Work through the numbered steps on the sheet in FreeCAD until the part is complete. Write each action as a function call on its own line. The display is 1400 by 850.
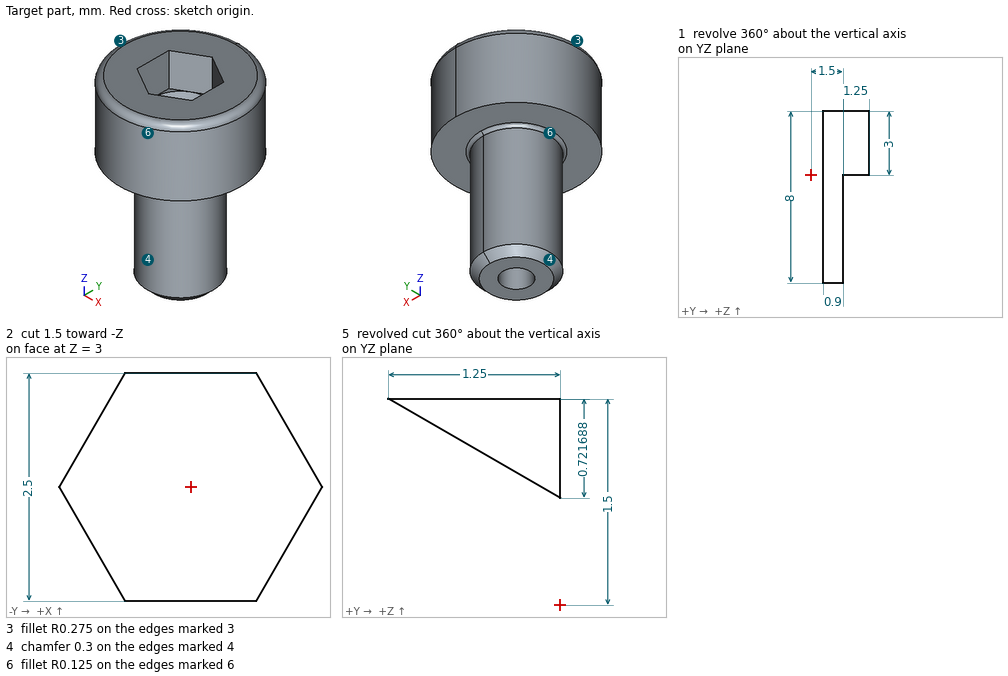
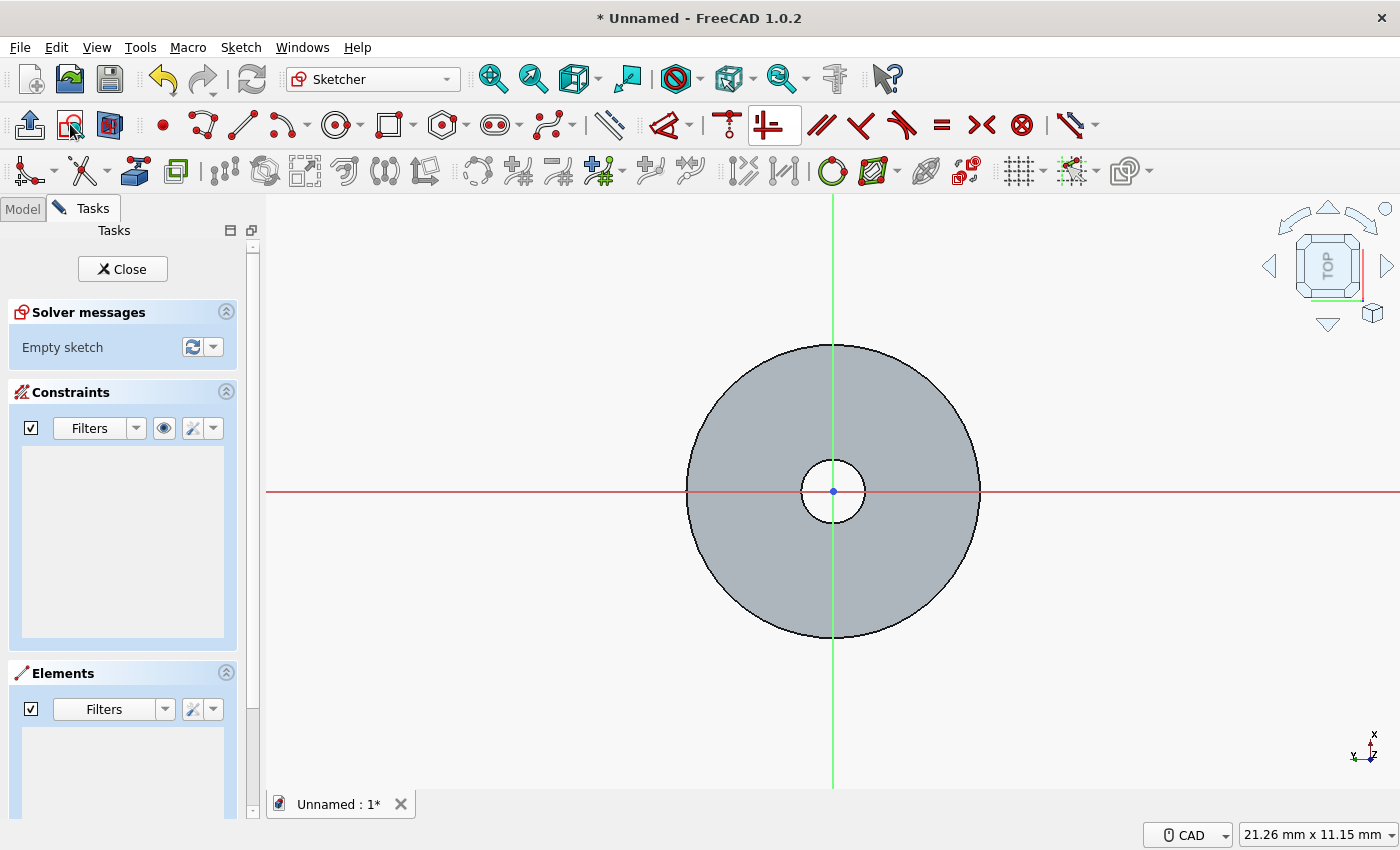
scroll(873, 492, up, 5)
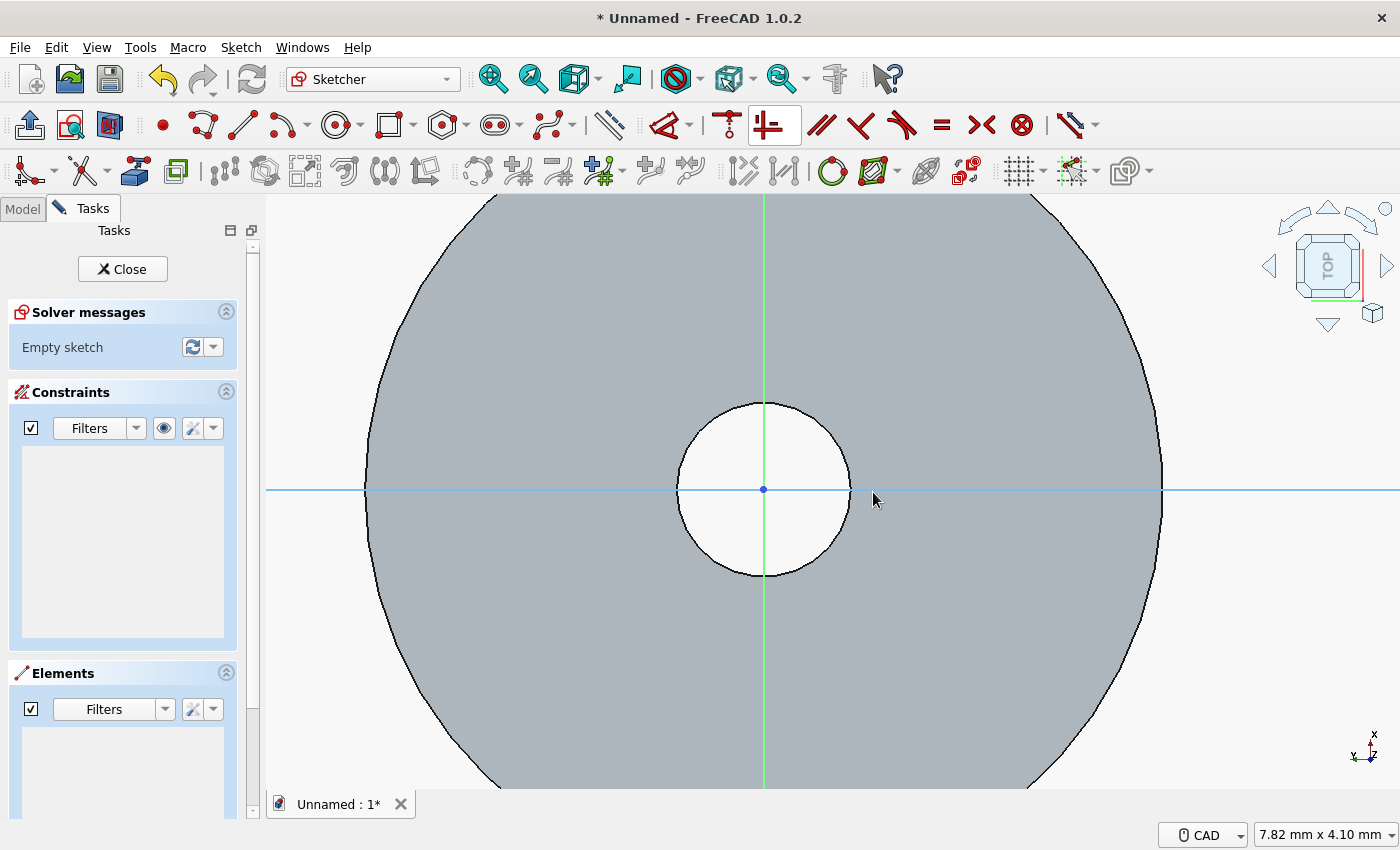
click(442, 126)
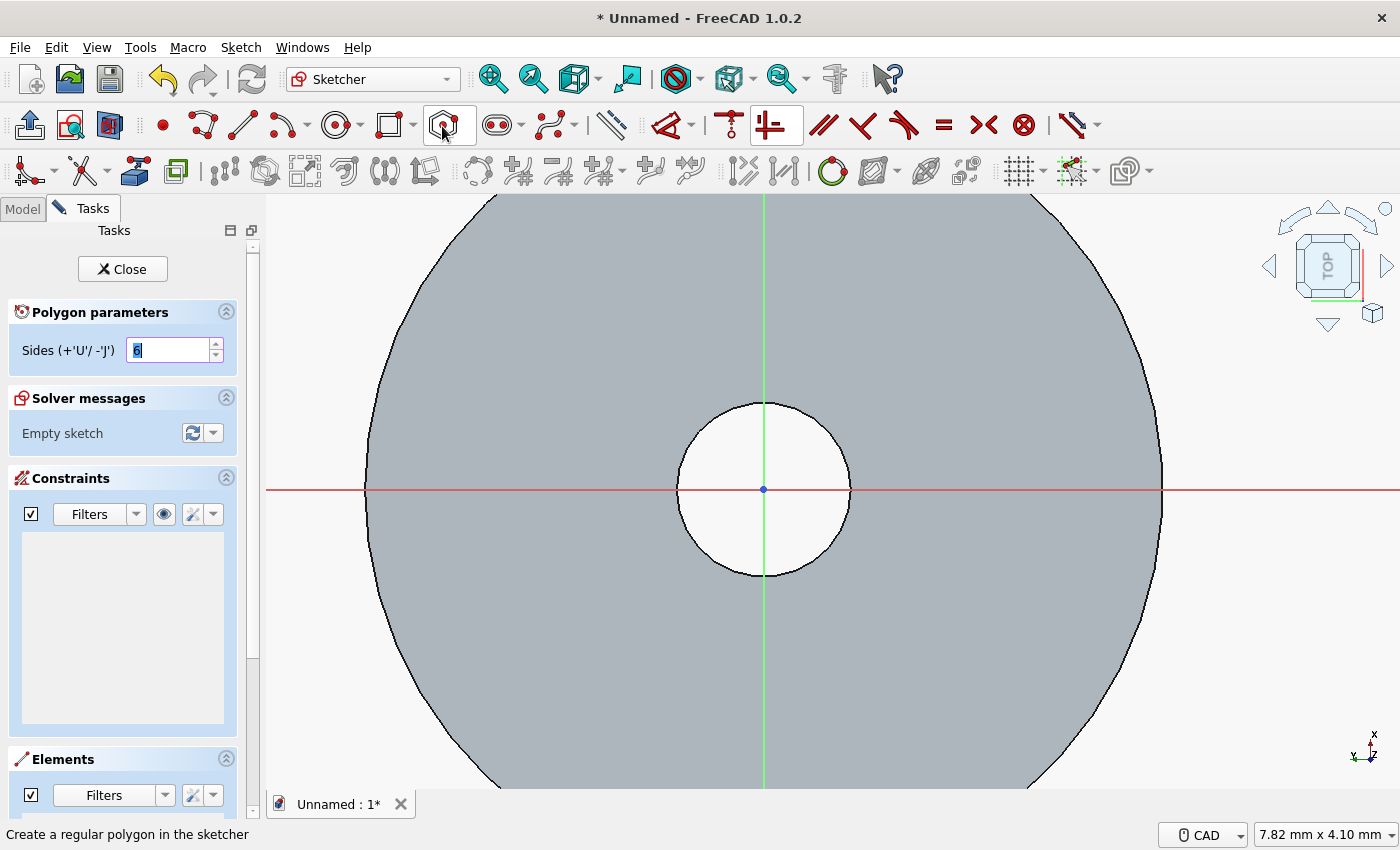
click(764, 490)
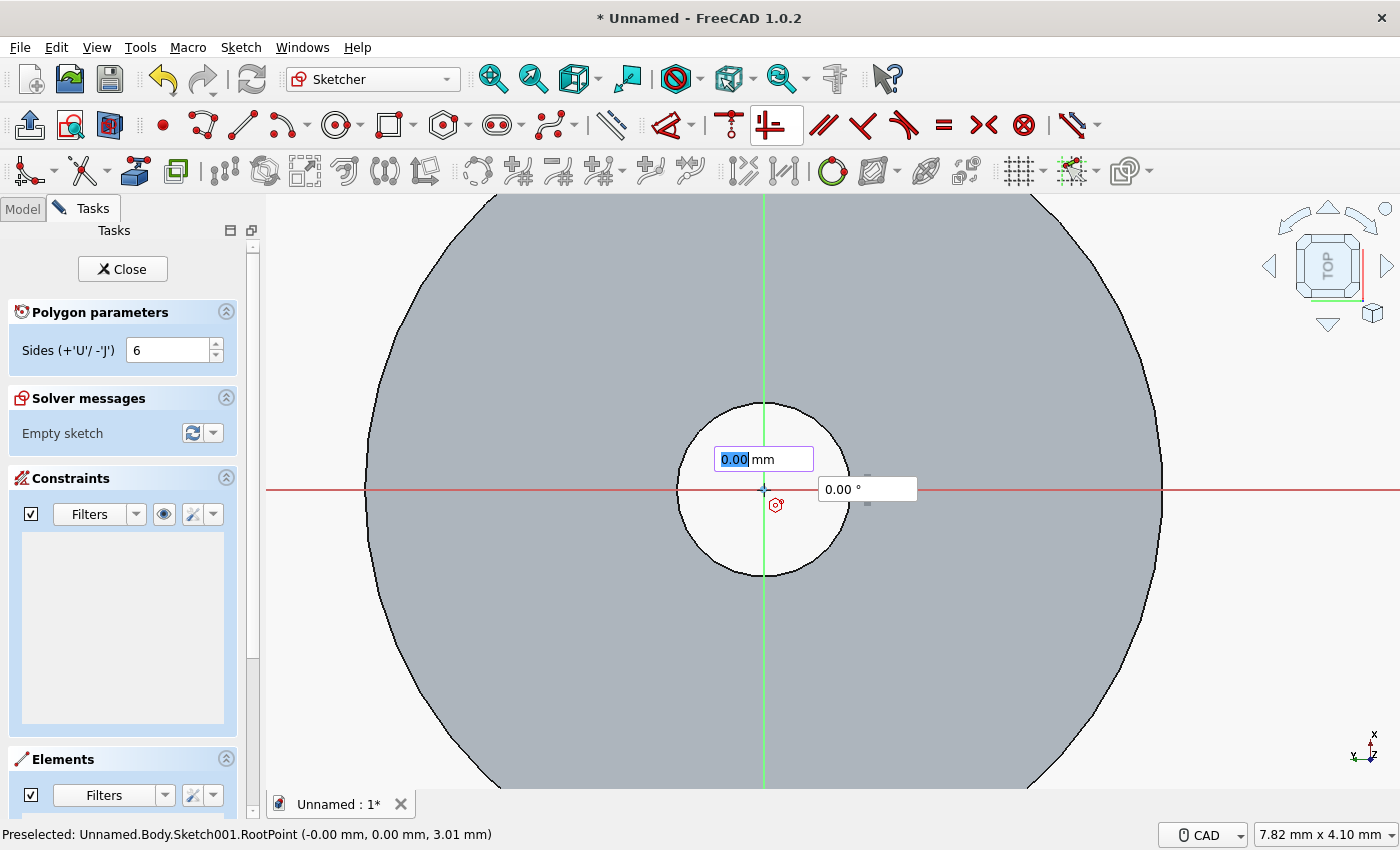
click(554, 490)
right_click(554, 490)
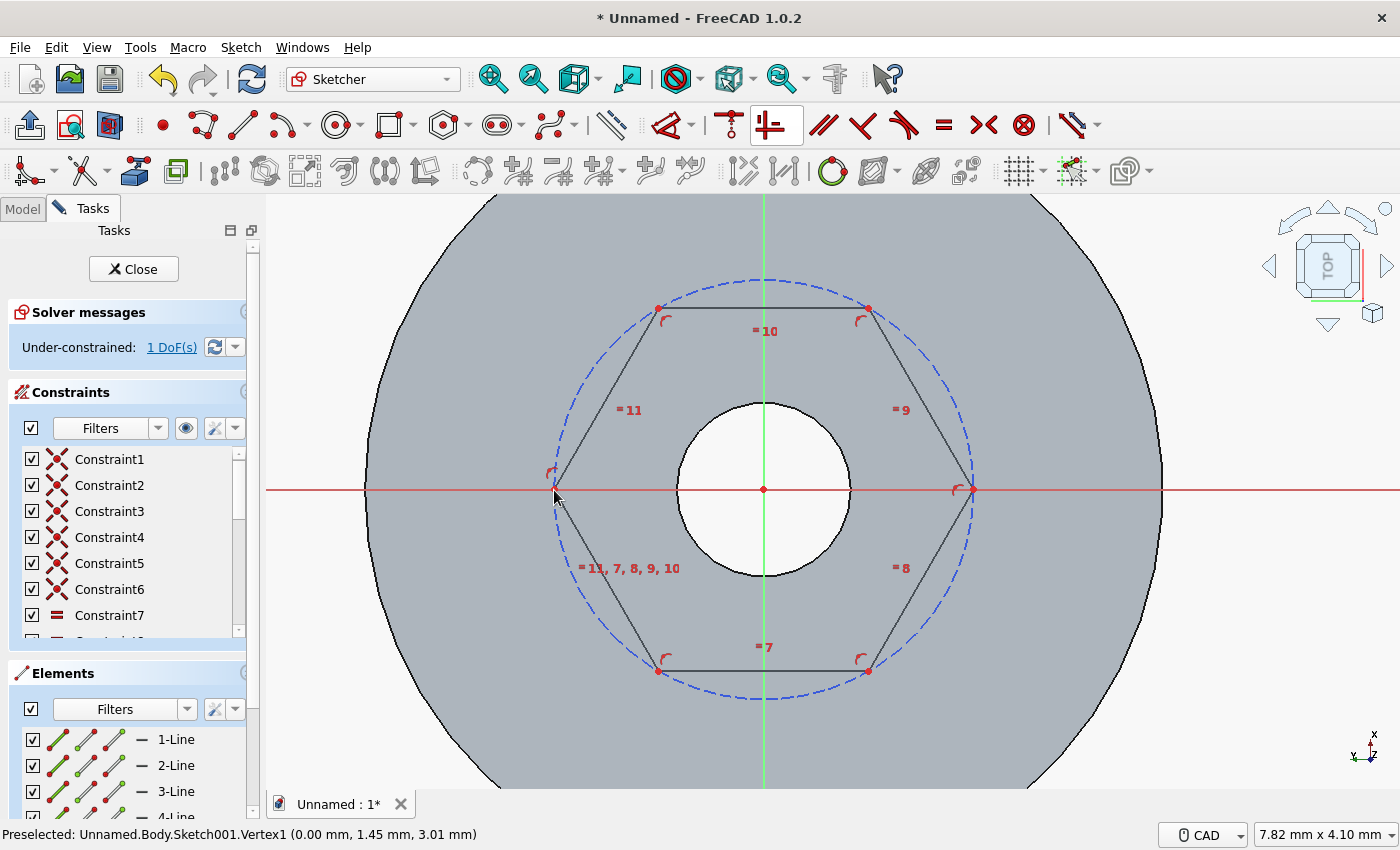
click(666, 126)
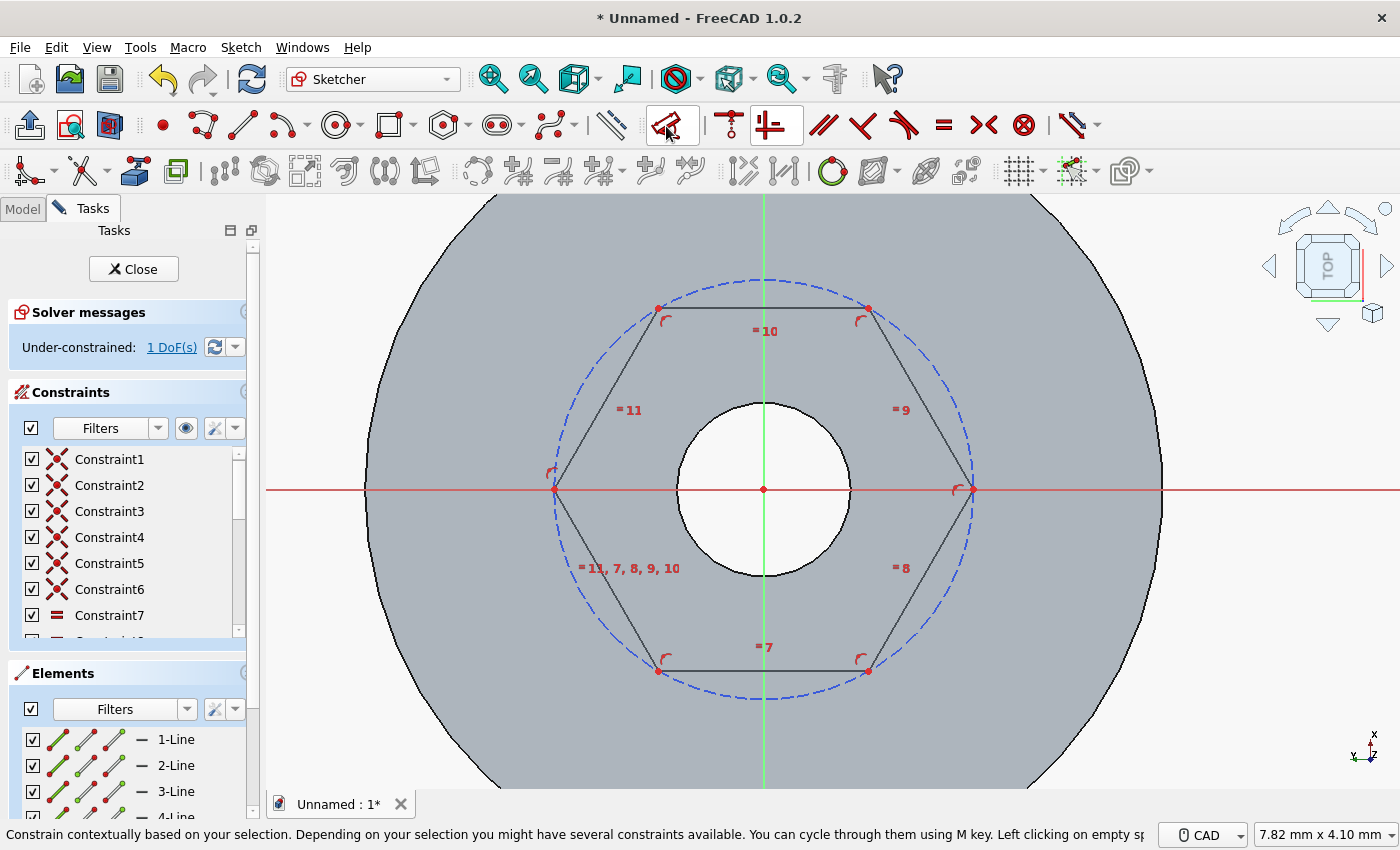
click(659, 671)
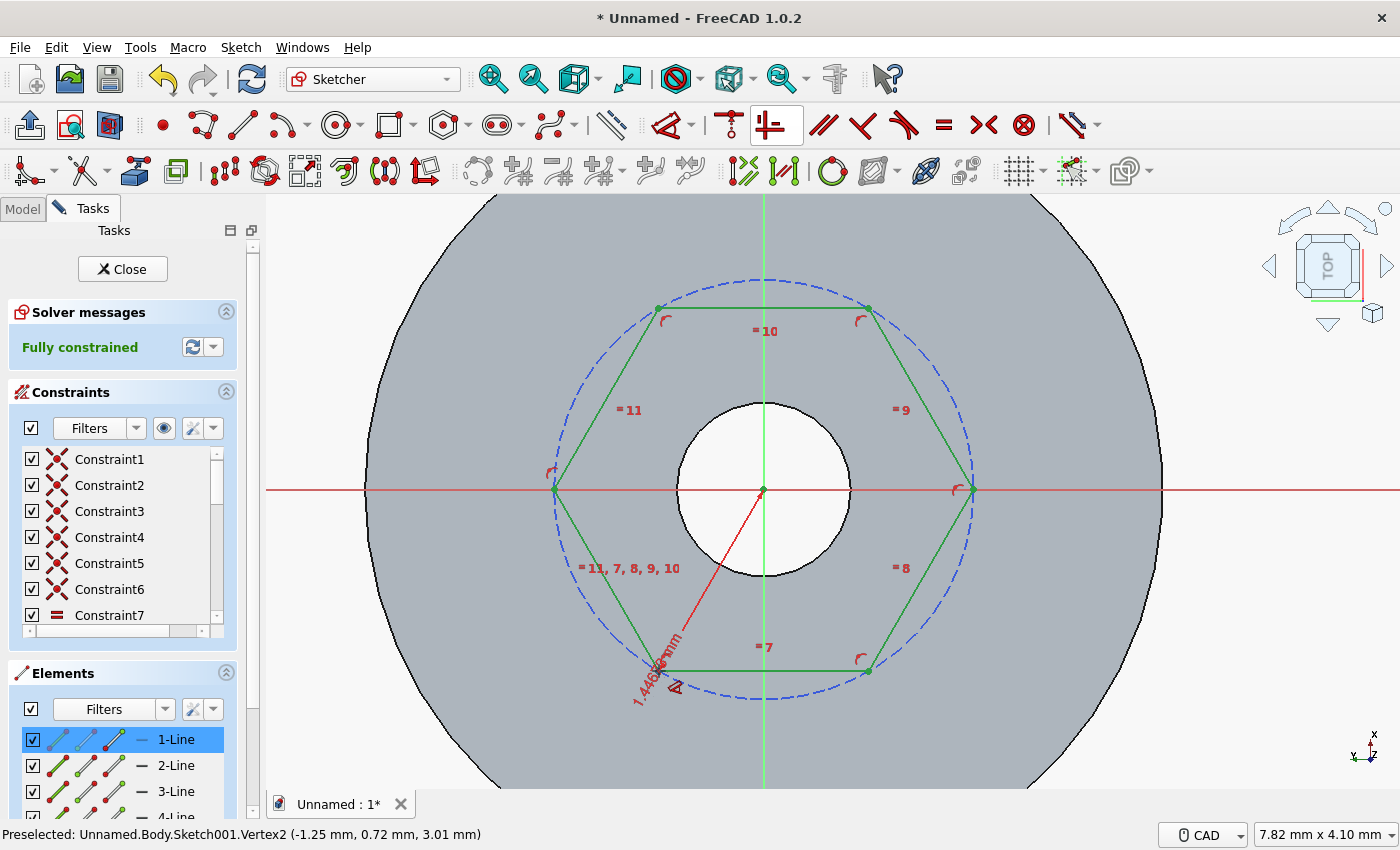
click(869, 308)
click(903, 406)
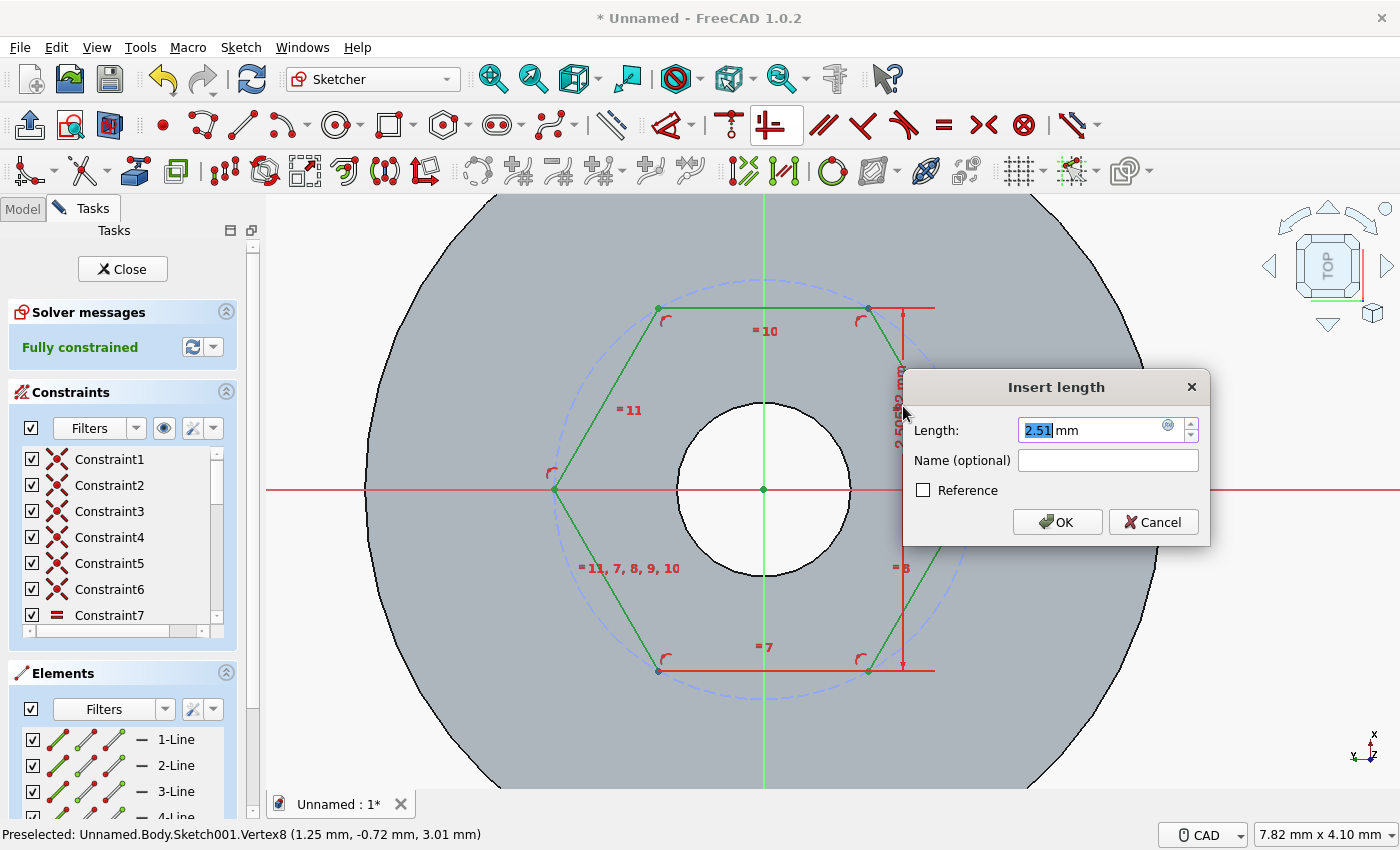
text(2.5)
key(Return)
key(Escape)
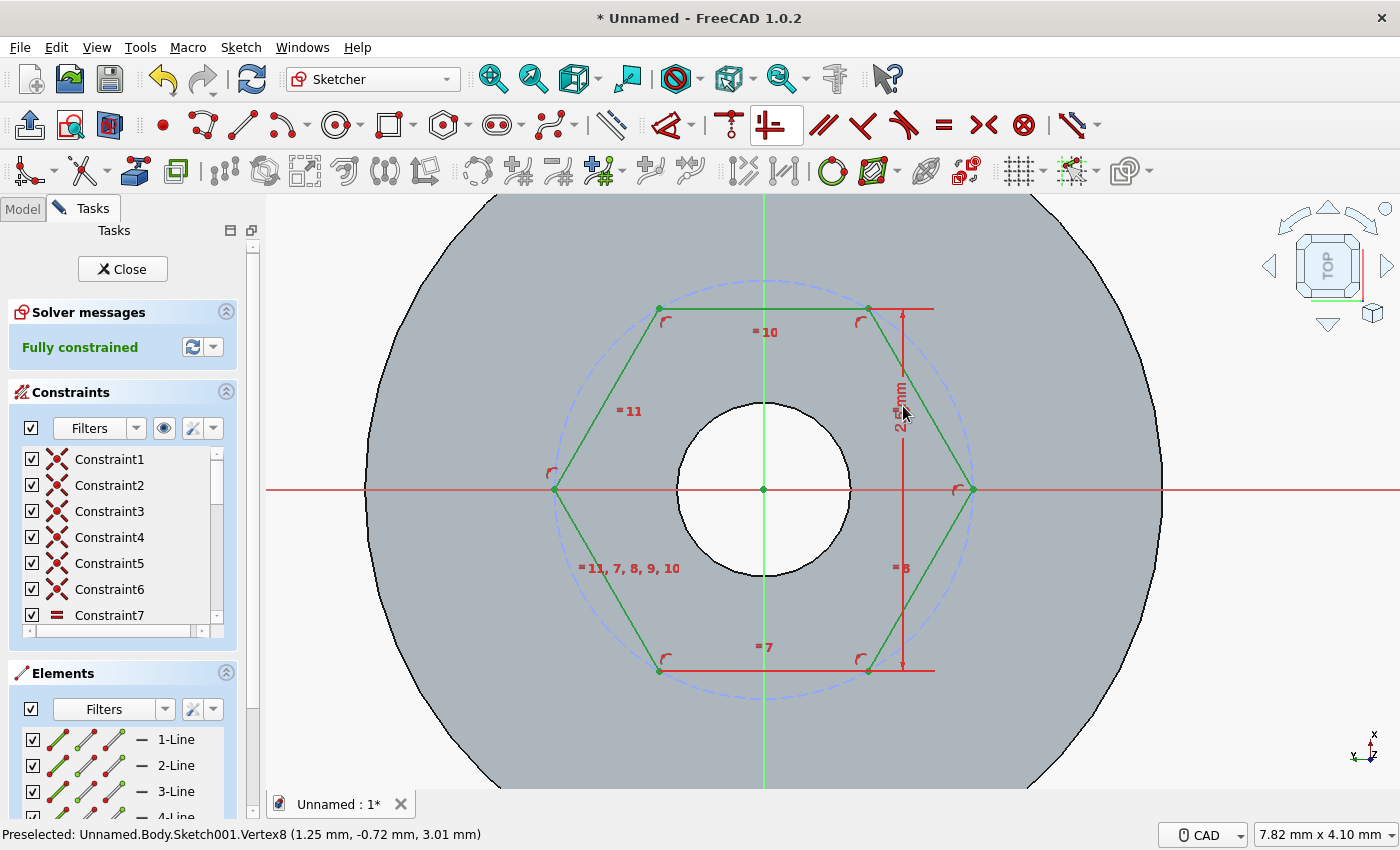
click(123, 269)